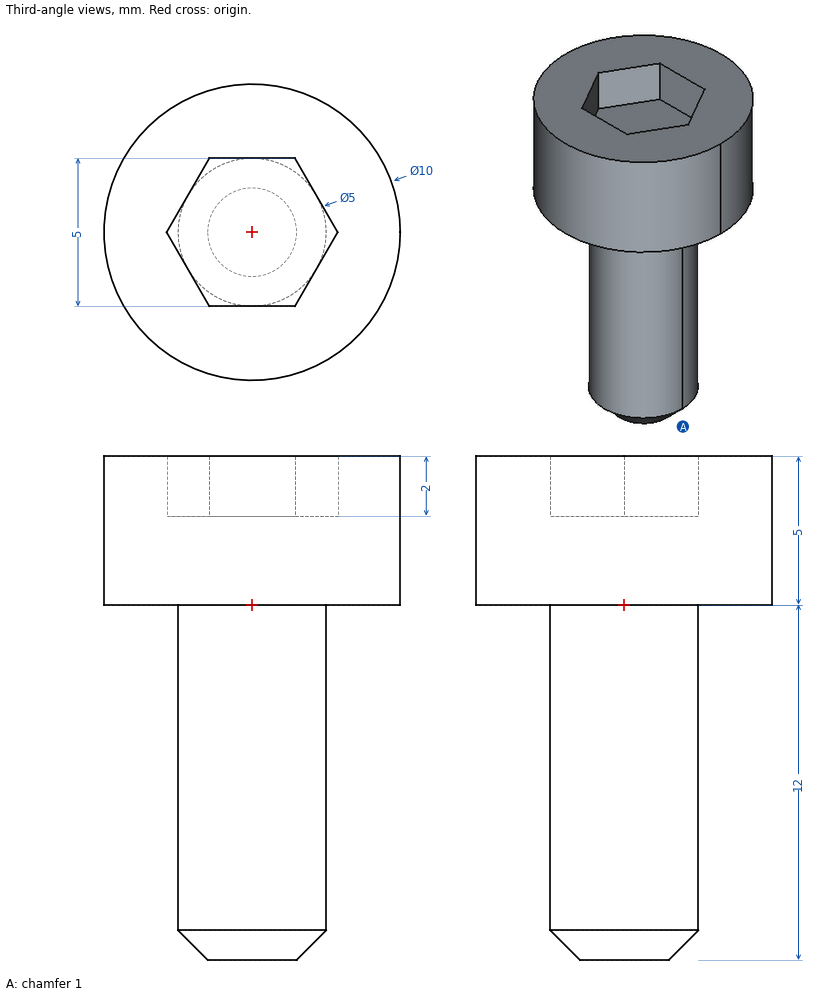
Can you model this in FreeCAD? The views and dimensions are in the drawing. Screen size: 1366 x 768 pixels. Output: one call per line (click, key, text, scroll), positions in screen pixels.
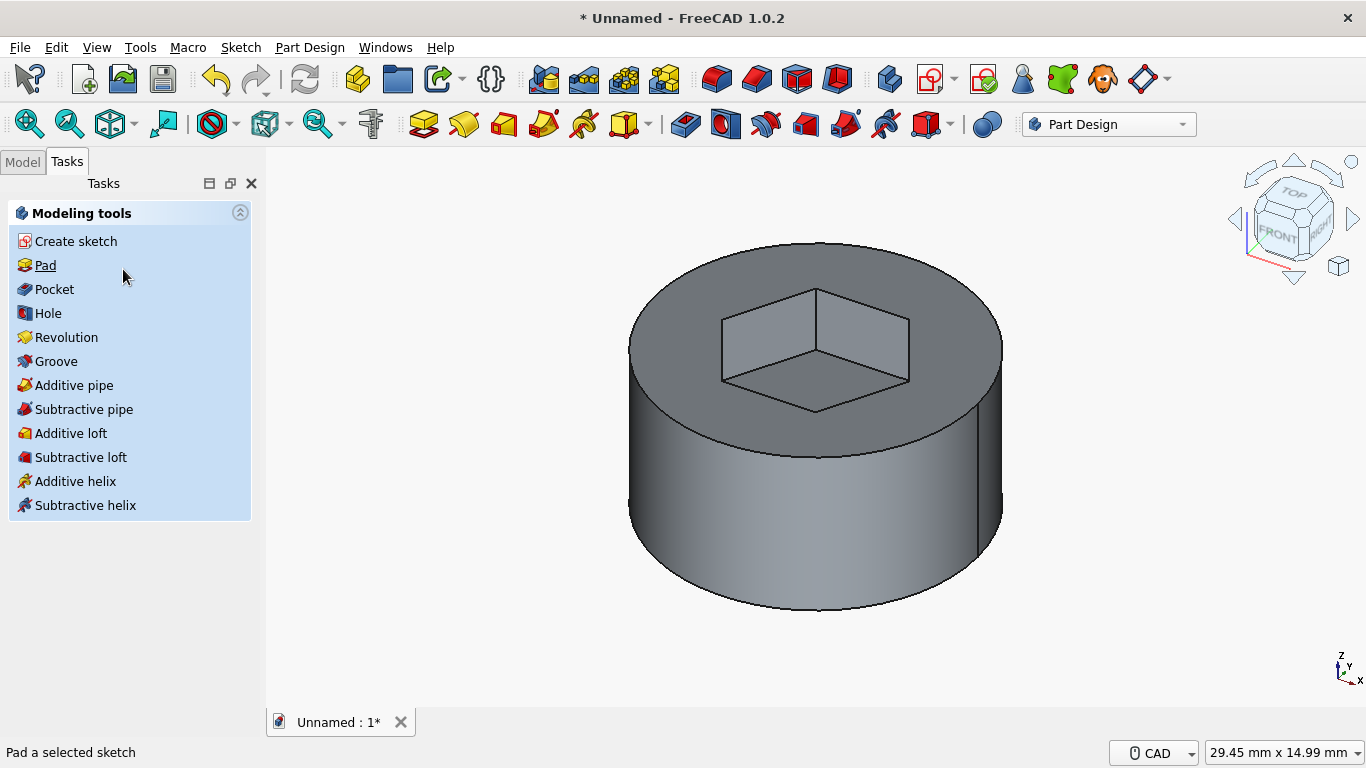
click(424, 124)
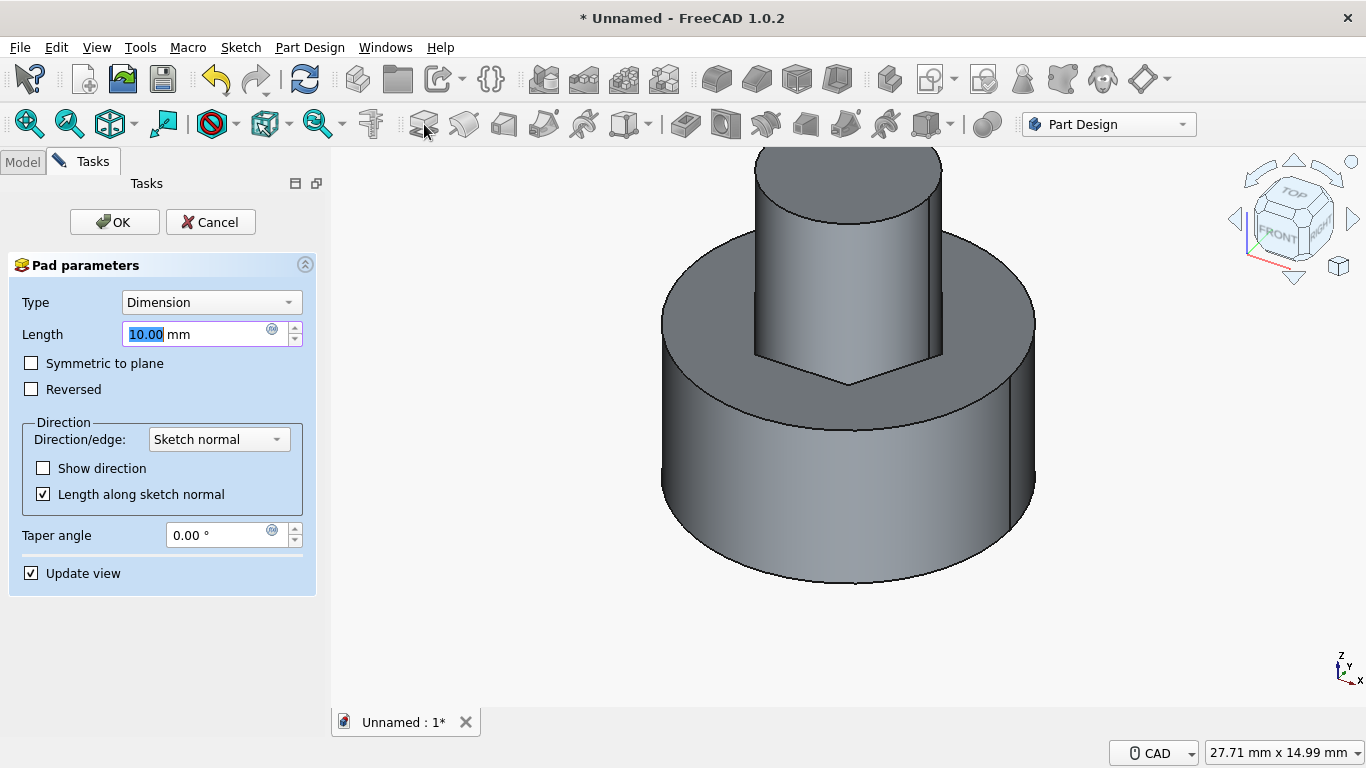
text(12)
key(Tab)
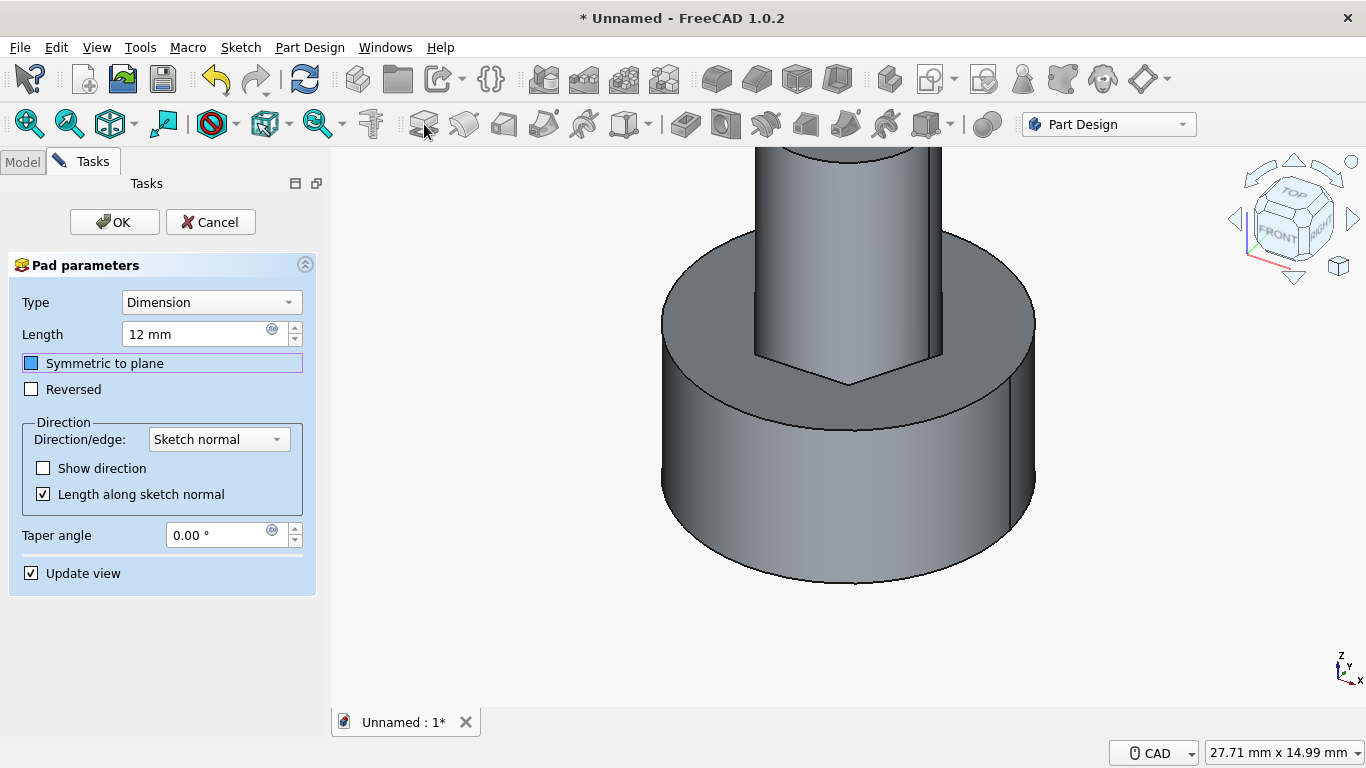
click(30, 389)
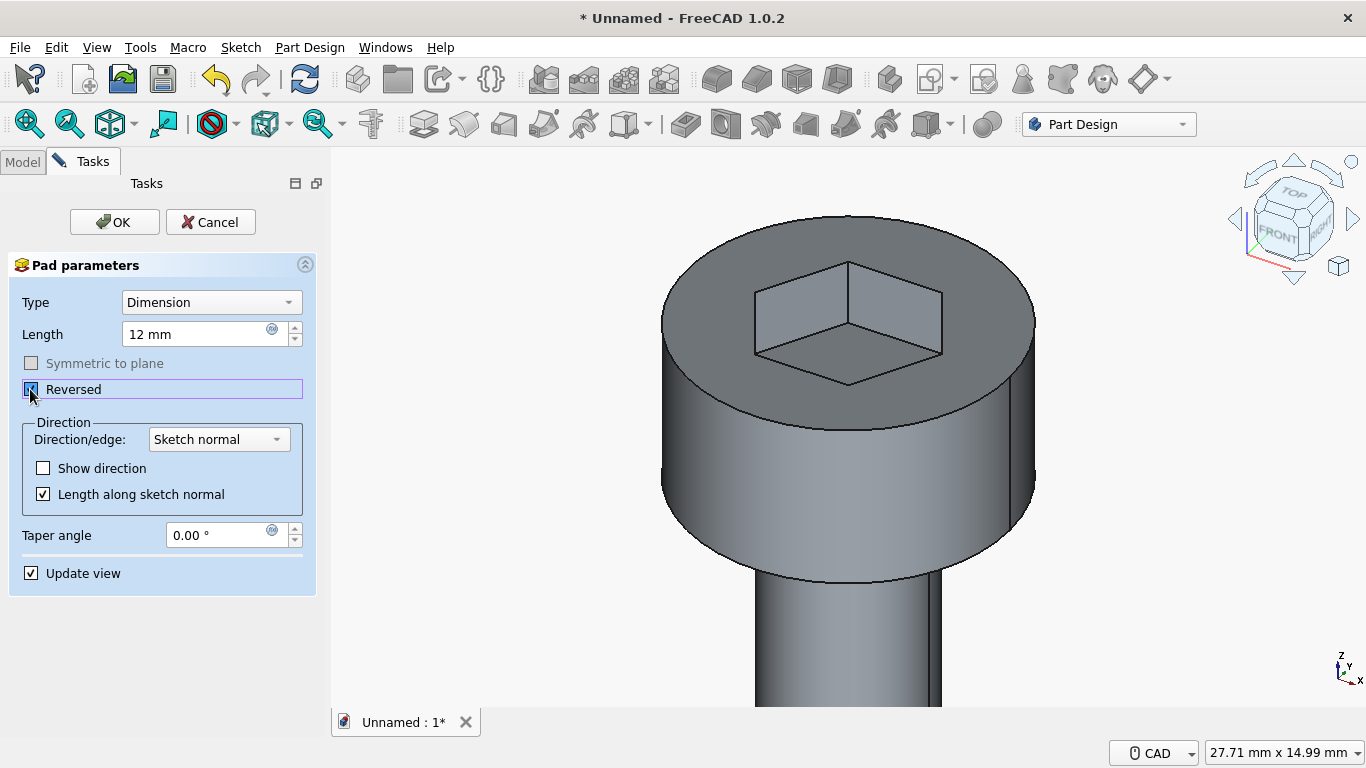
click(115, 222)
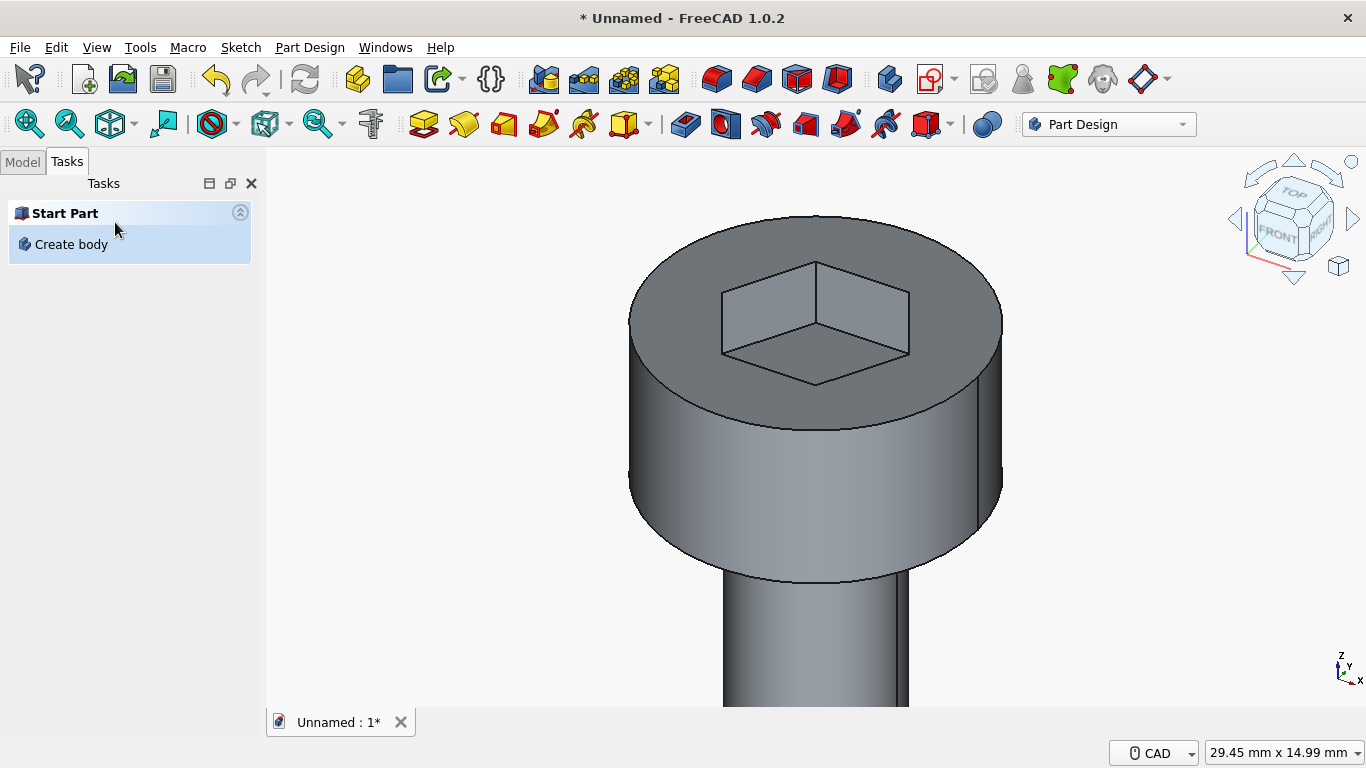
key(v)
key(f)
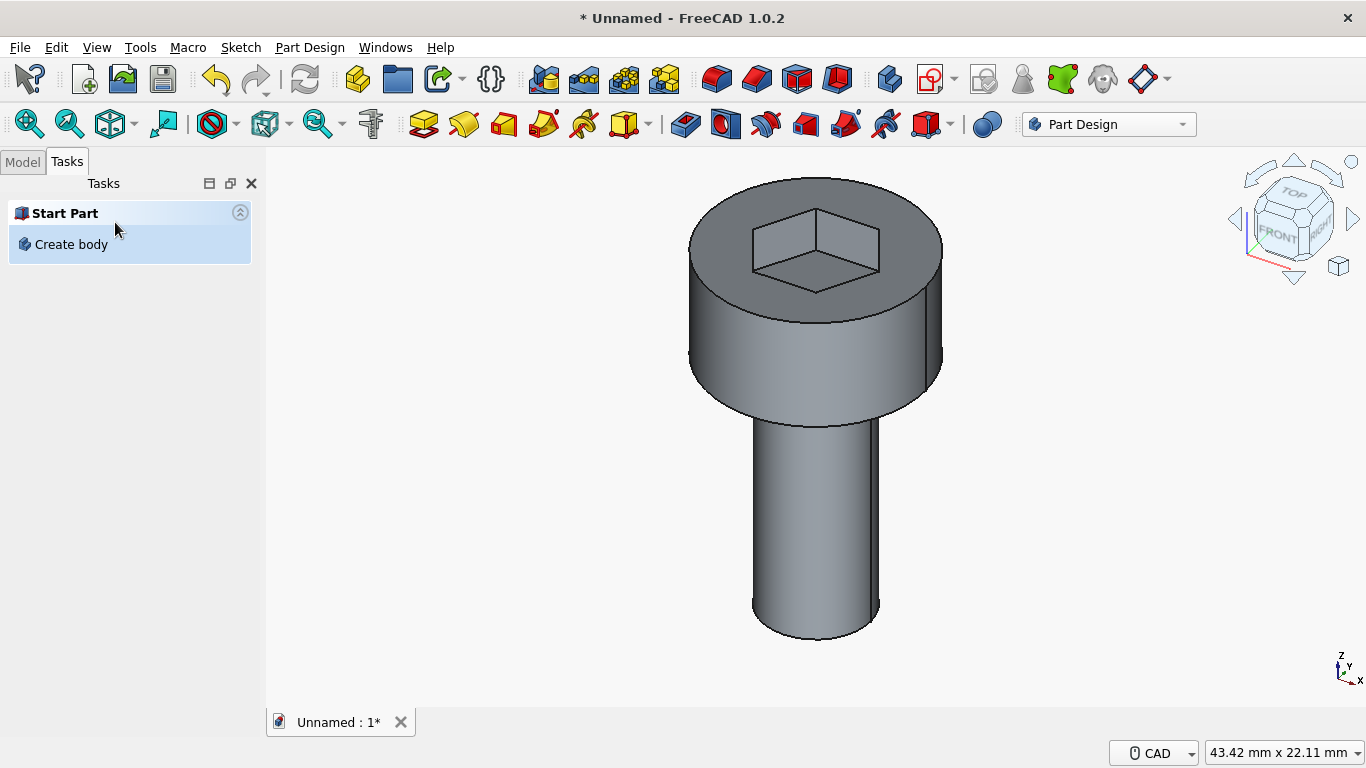
key(0)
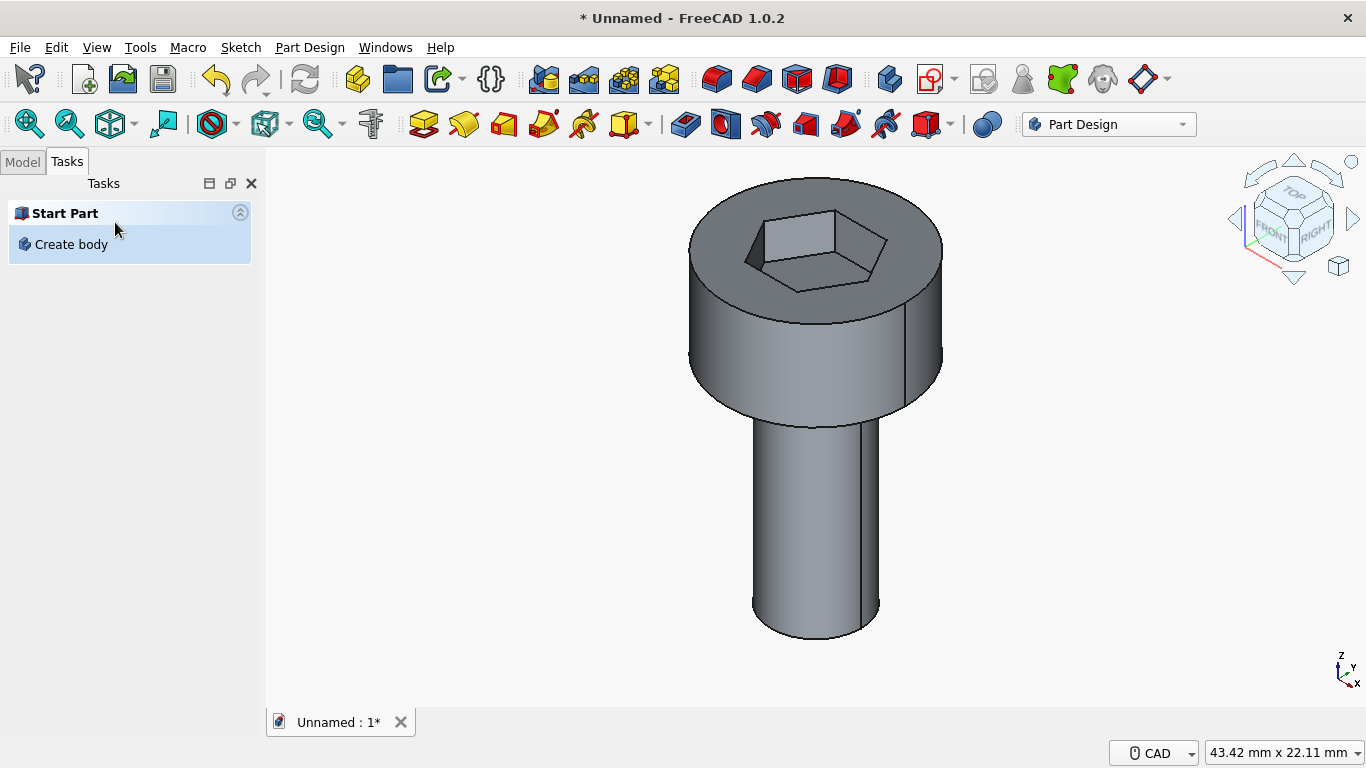
key(2)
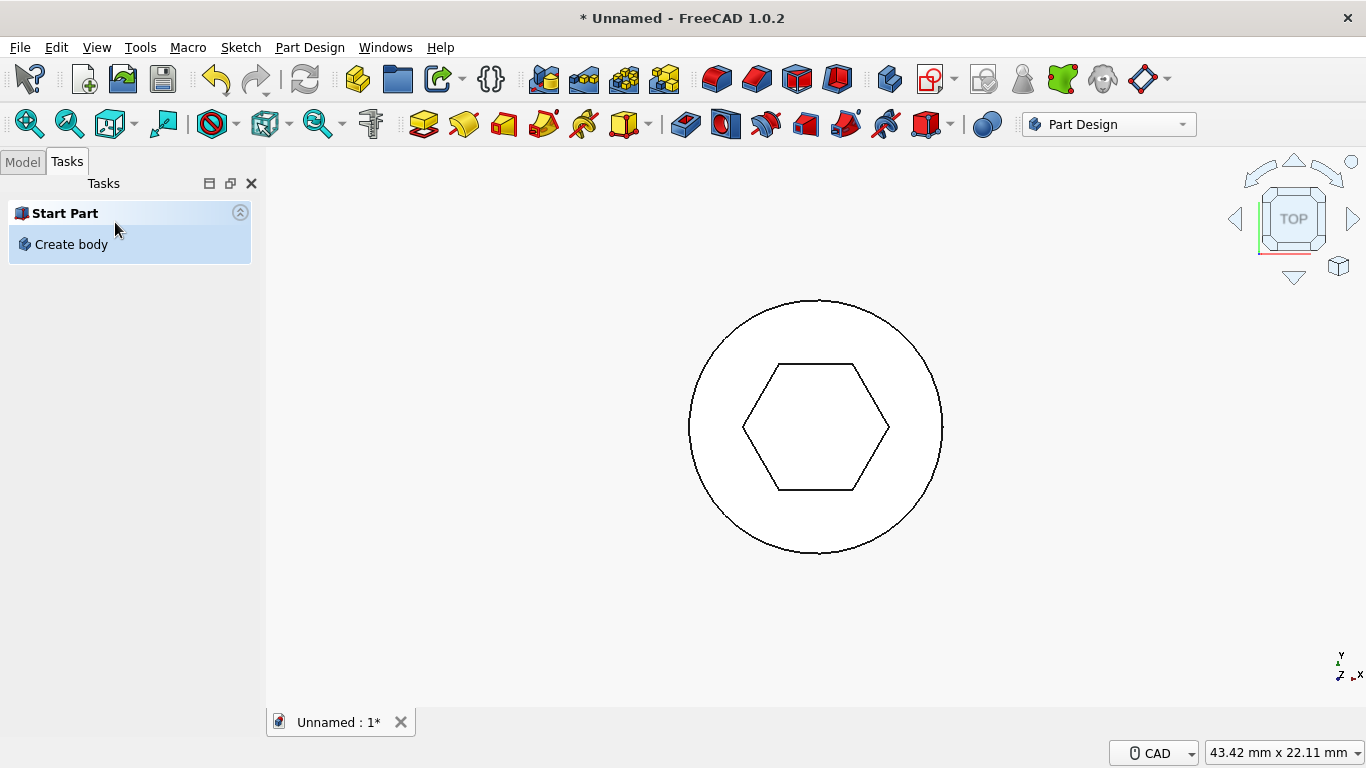
key(1)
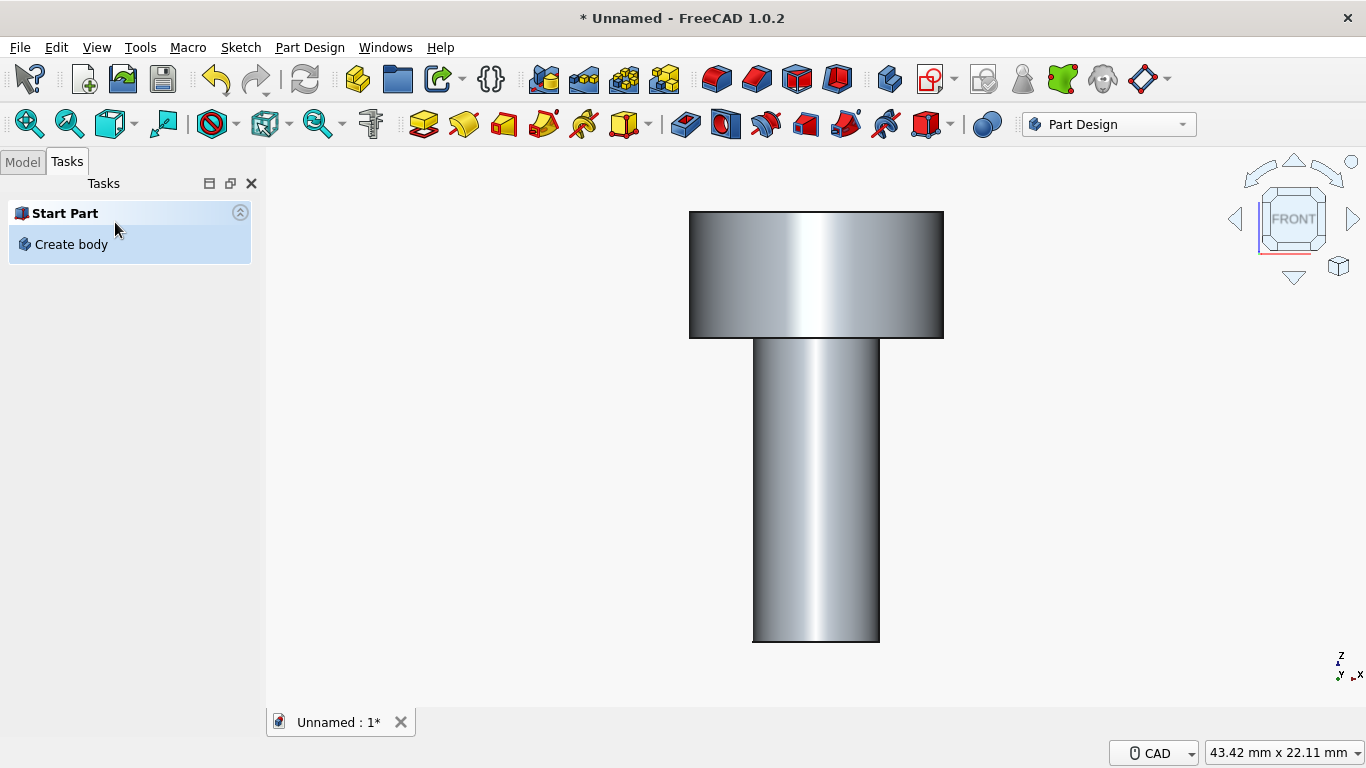
click(765, 641)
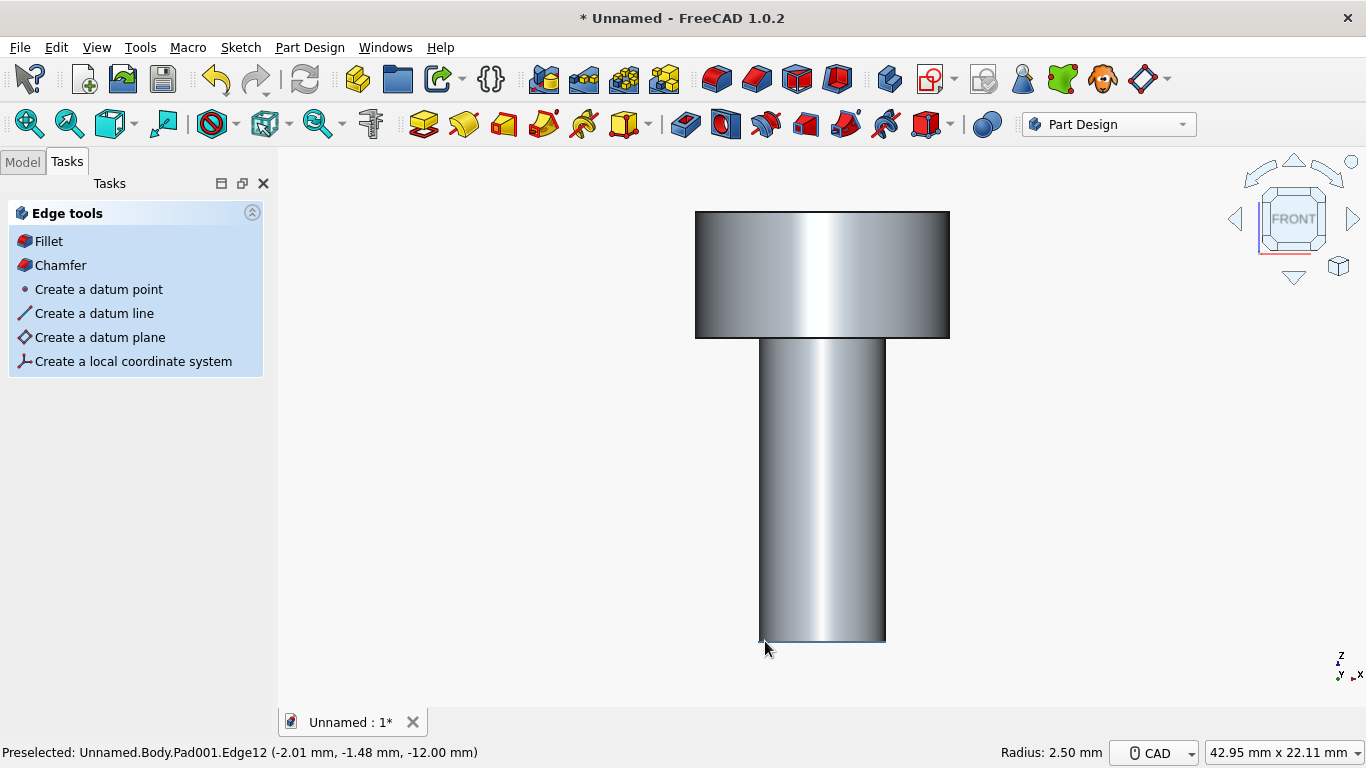
click(758, 80)